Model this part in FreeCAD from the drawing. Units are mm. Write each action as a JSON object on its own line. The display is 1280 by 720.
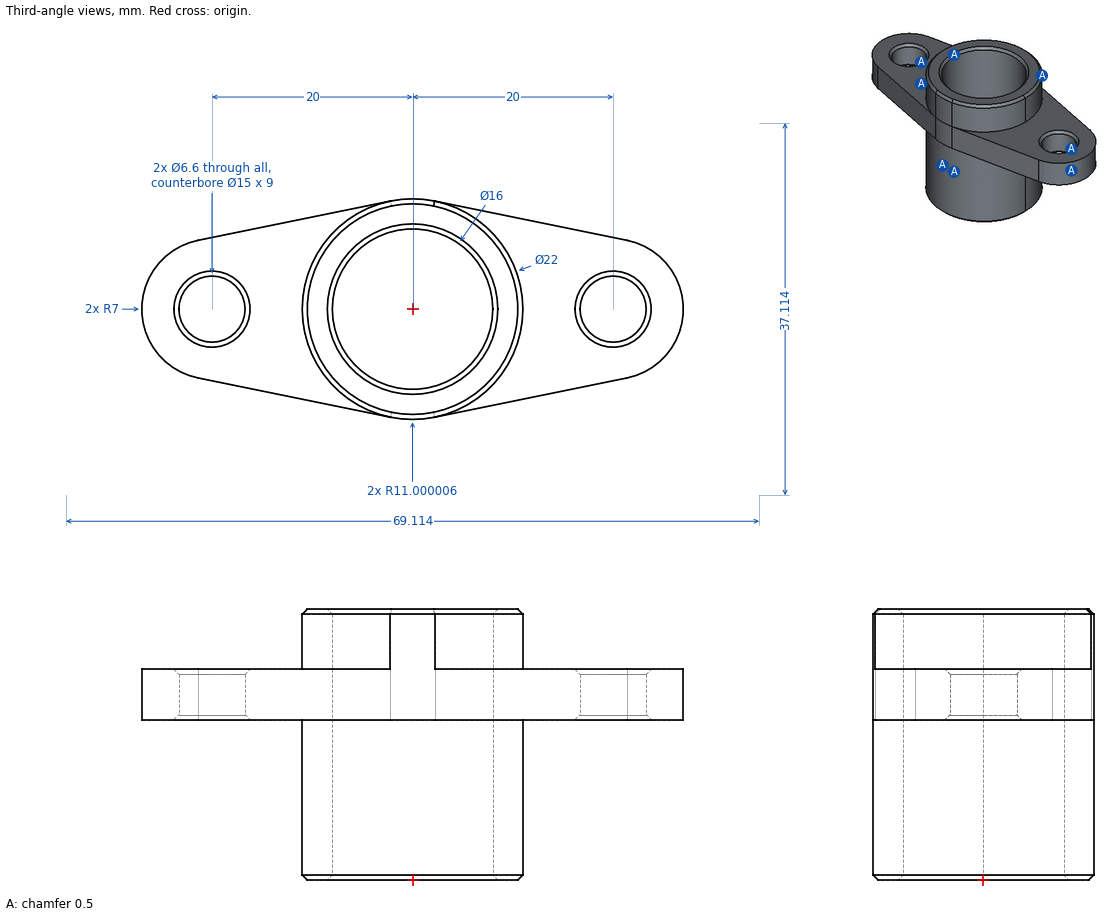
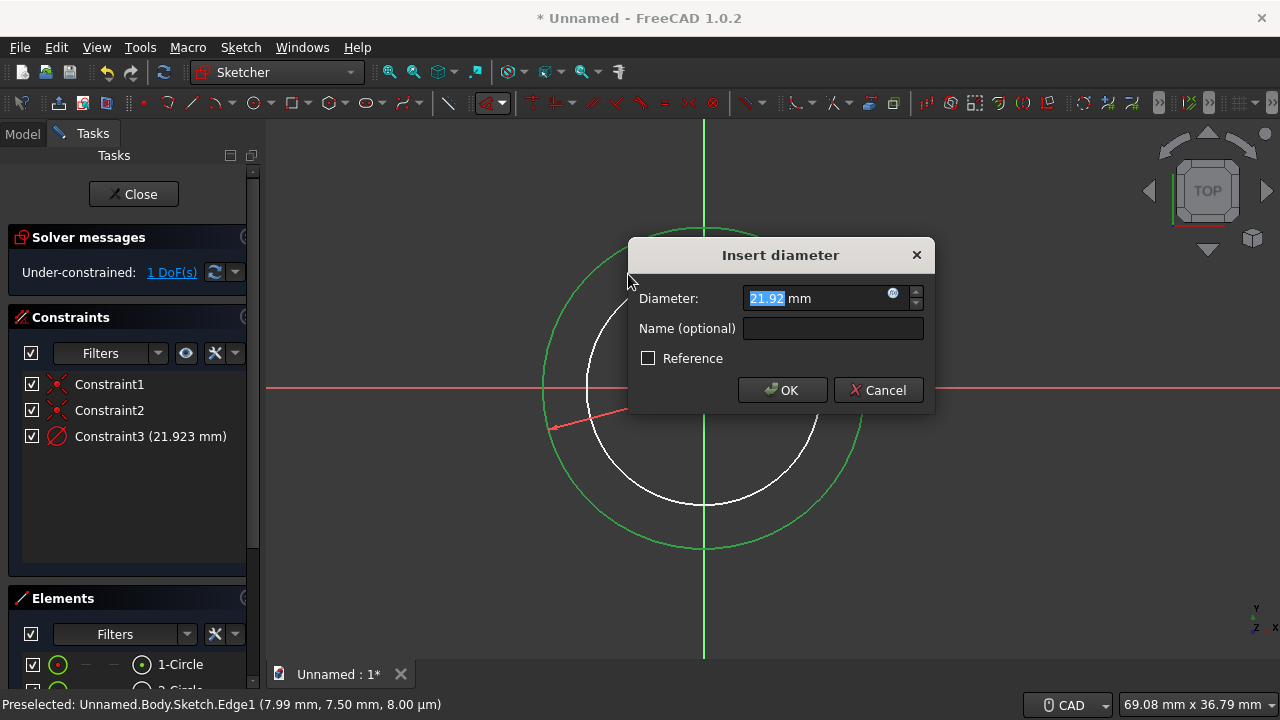
{"action": "type", "text": "22"}
{"action": "key", "text": "Return"}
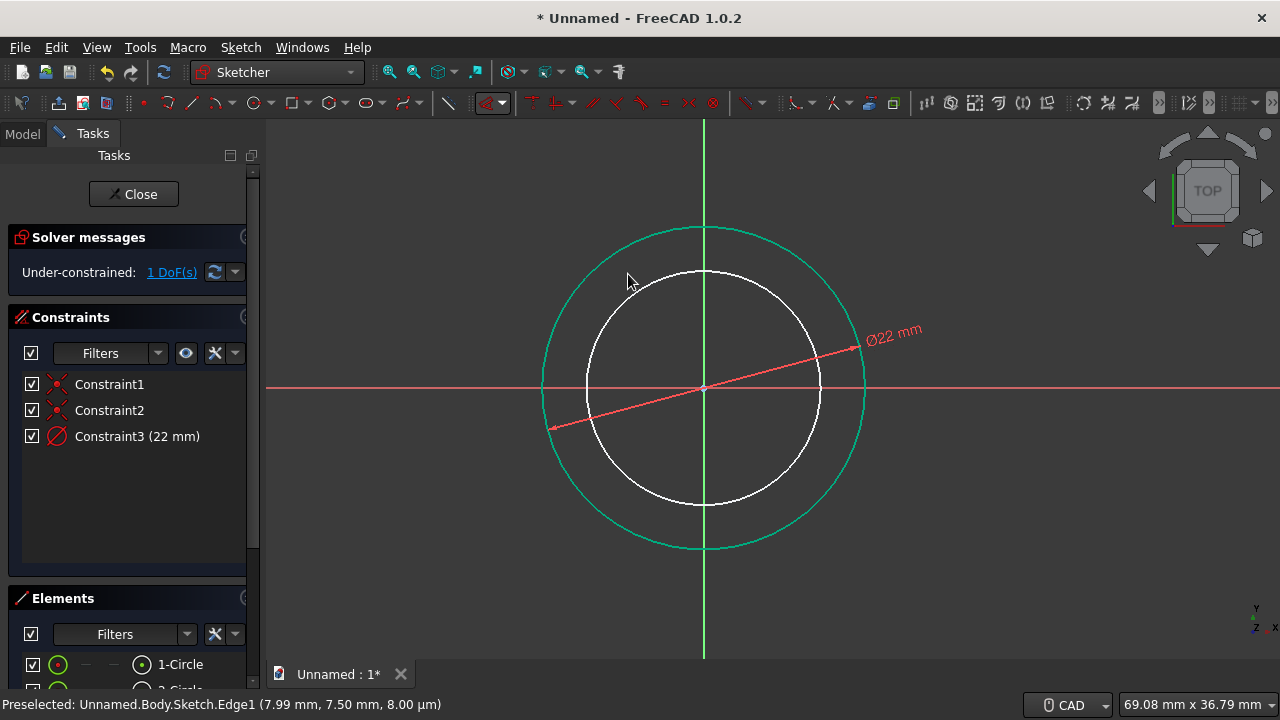
{"action": "left_click", "coordinate": [786, 305]}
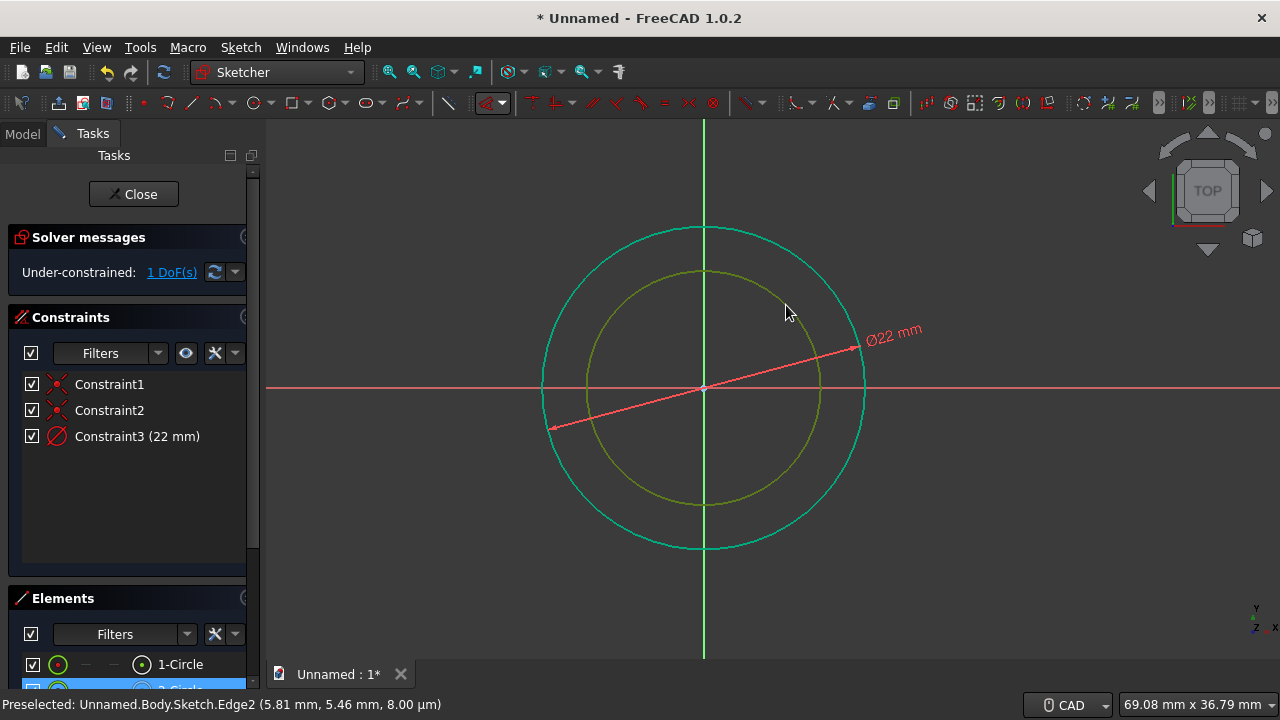
{"action": "key", "text": "k o"}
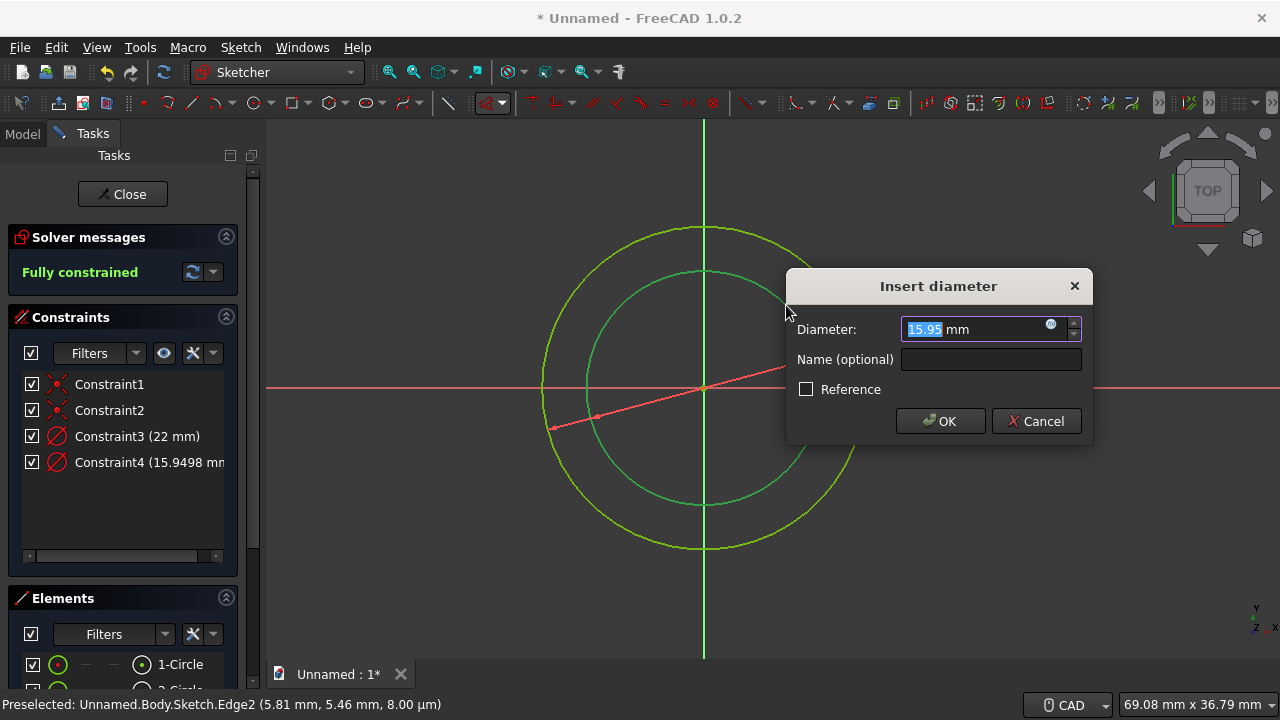
{"action": "type", "text": "16"}
{"action": "key", "text": "Return"}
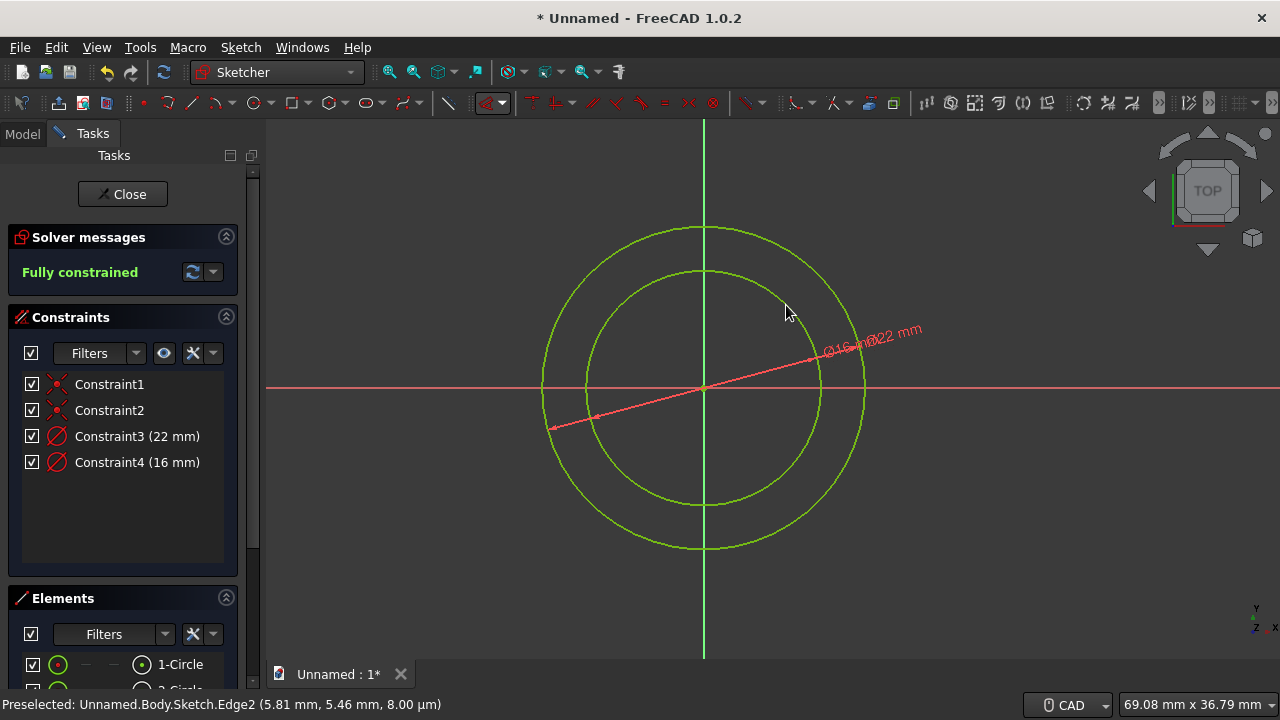
{"action": "left_click", "coordinate": [123, 194]}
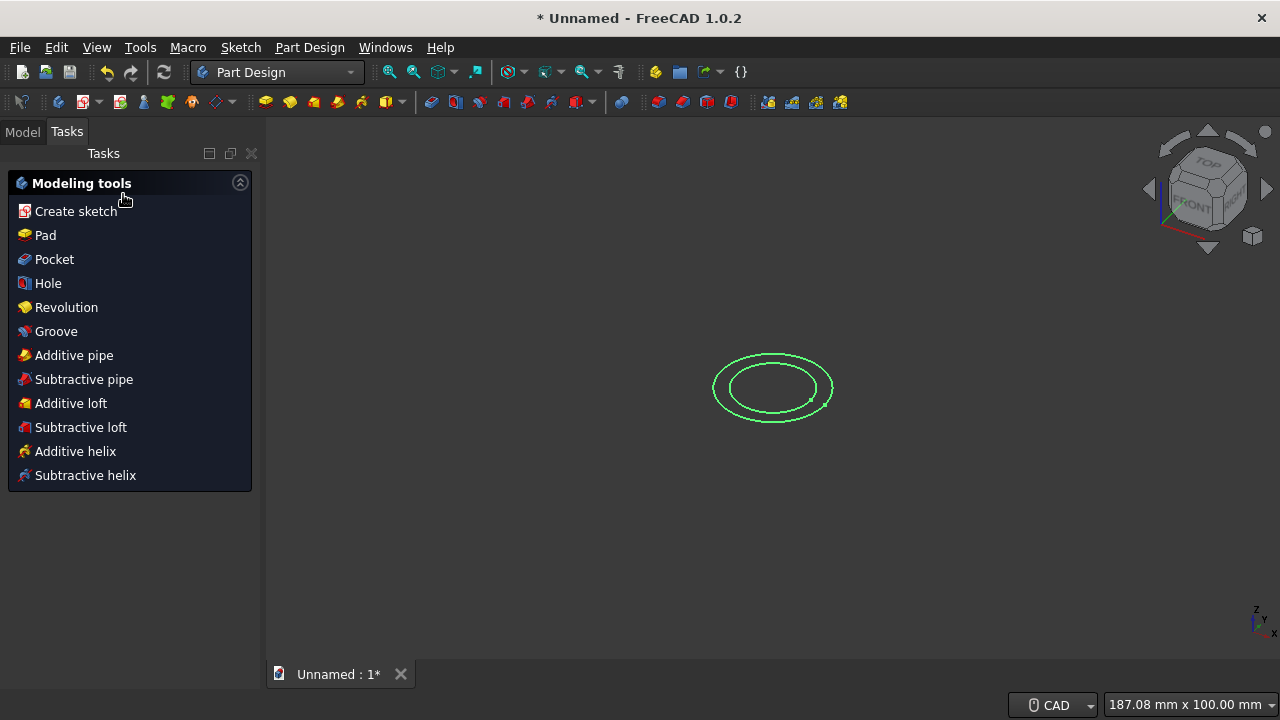
{"action": "left_click", "coordinate": [266, 102]}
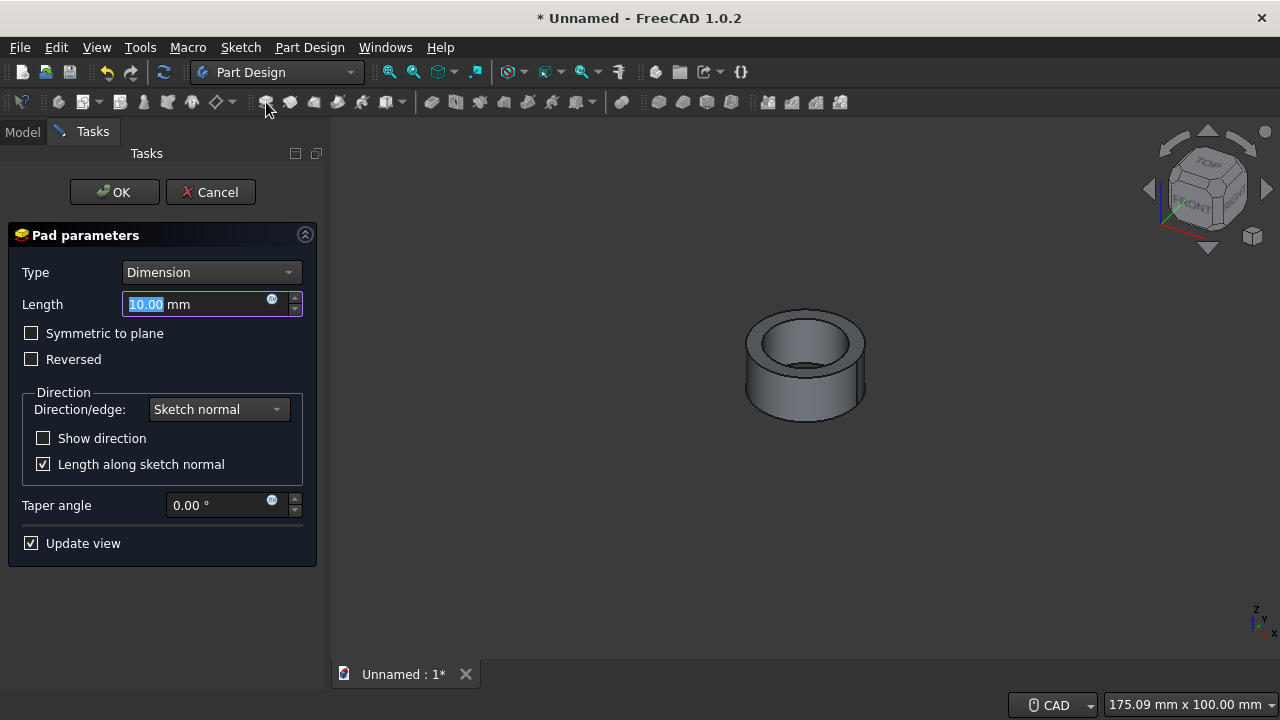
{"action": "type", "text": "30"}
{"action": "key", "text": "Tab"}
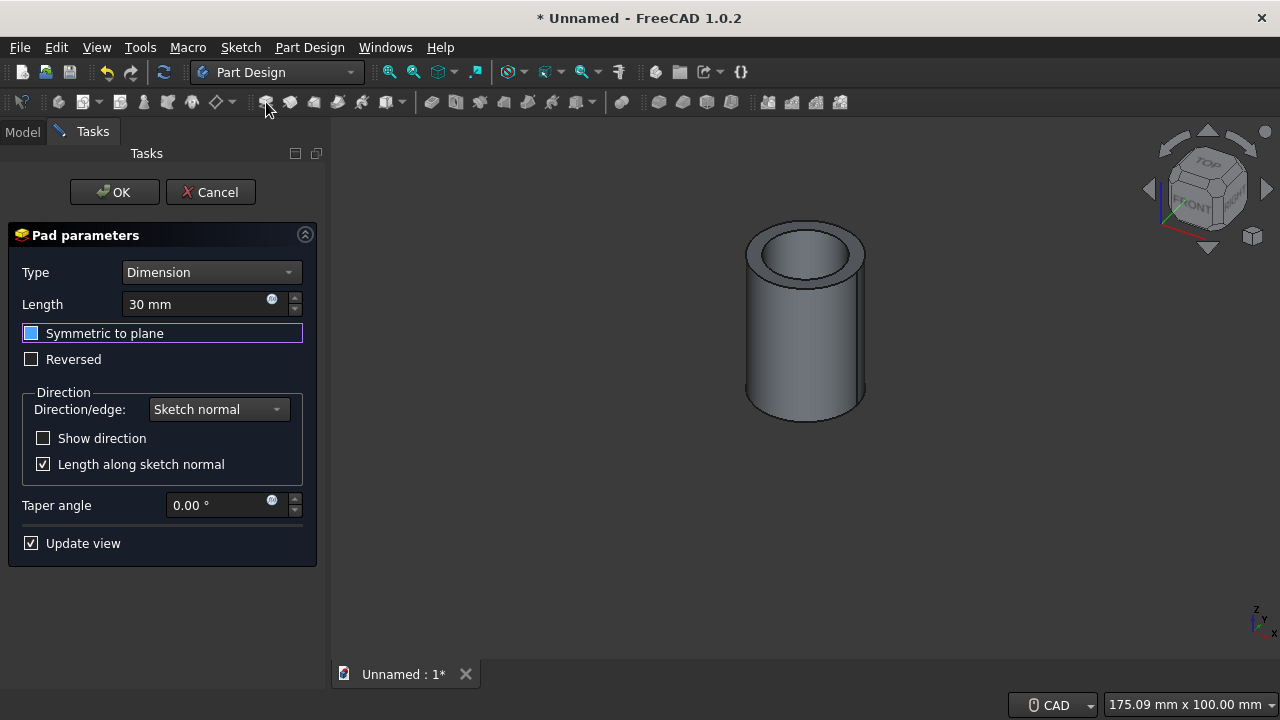
{"action": "left_click", "coordinate": [115, 192]}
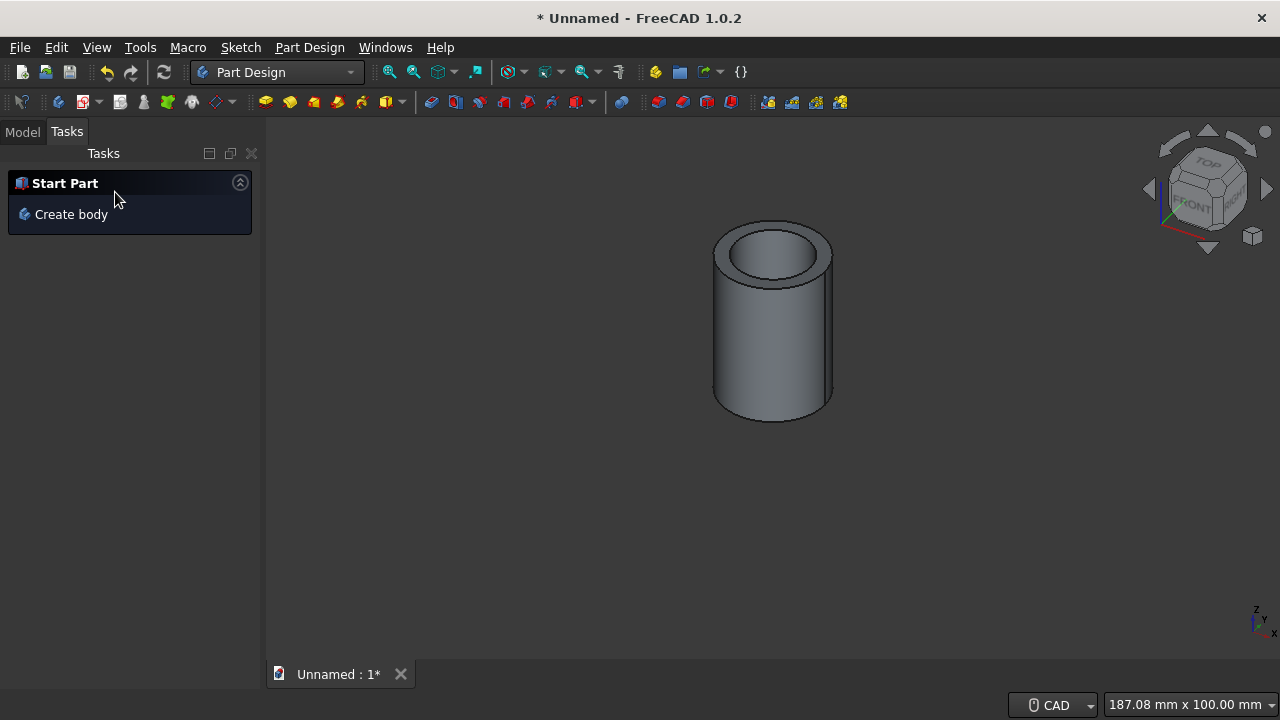
{"action": "left_click", "coordinate": [390, 72]}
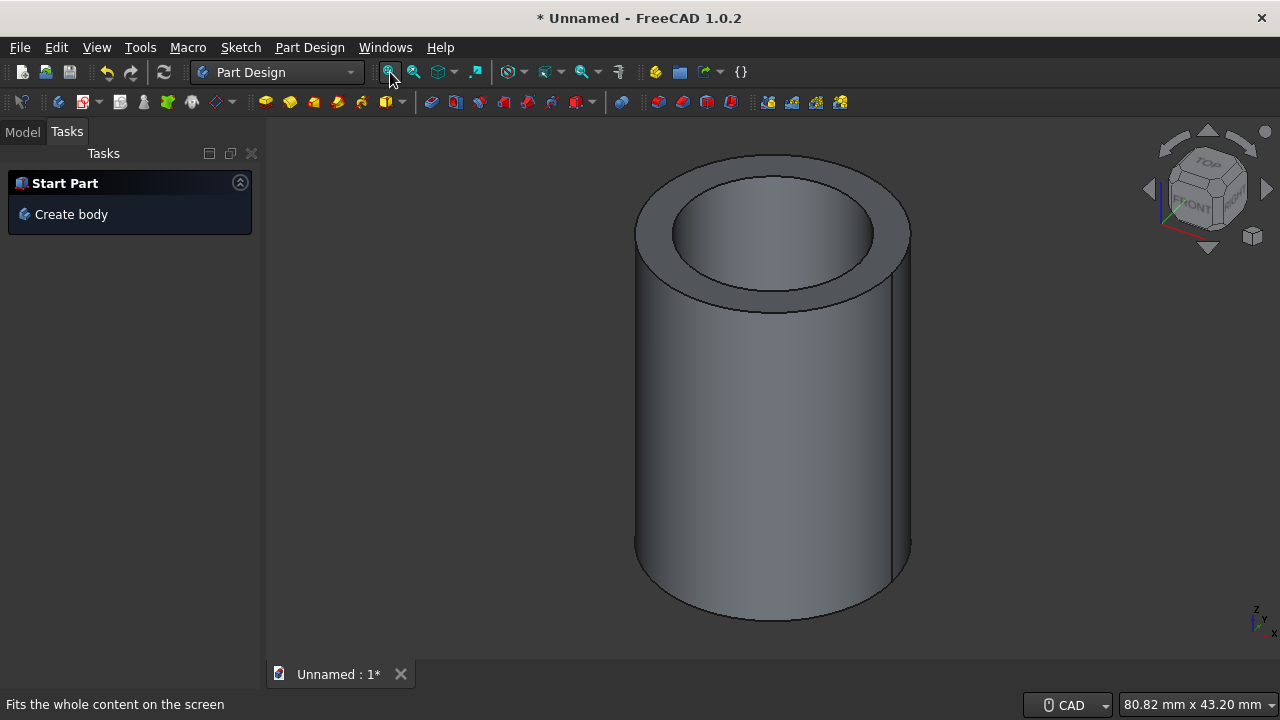
{"action": "left_click", "coordinate": [23, 131]}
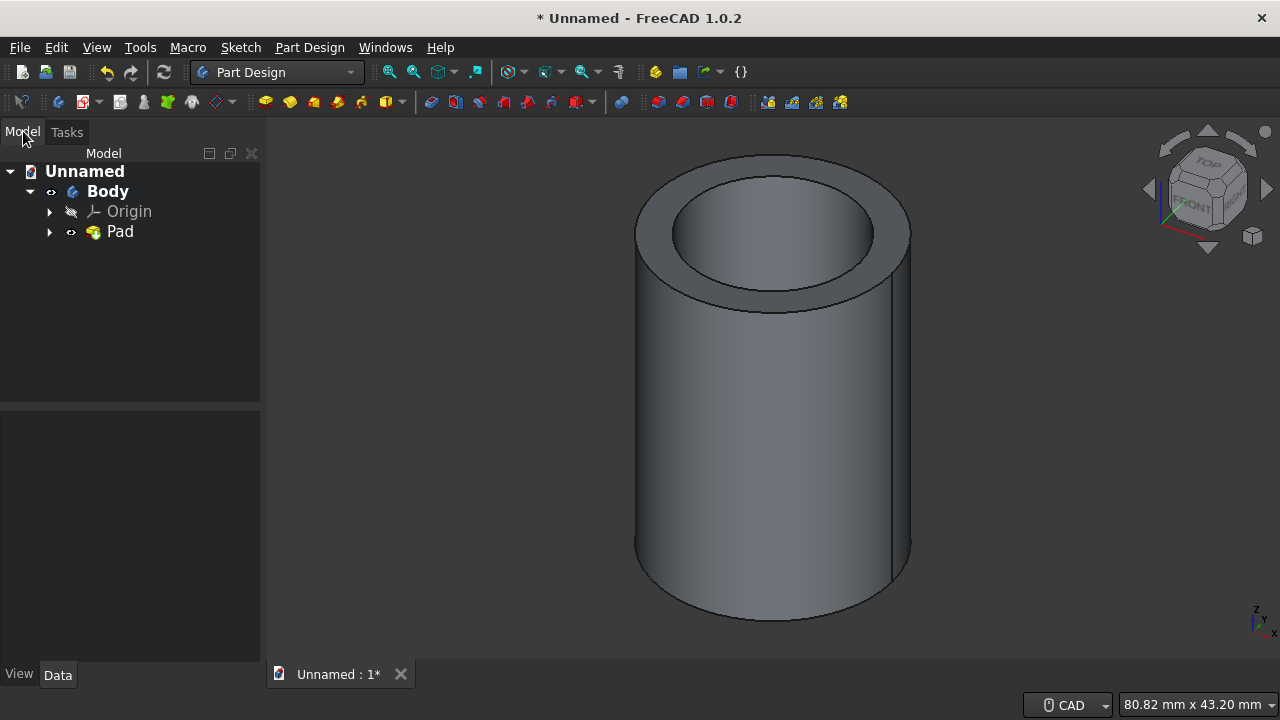
{"action": "left_click", "coordinate": [50, 212]}